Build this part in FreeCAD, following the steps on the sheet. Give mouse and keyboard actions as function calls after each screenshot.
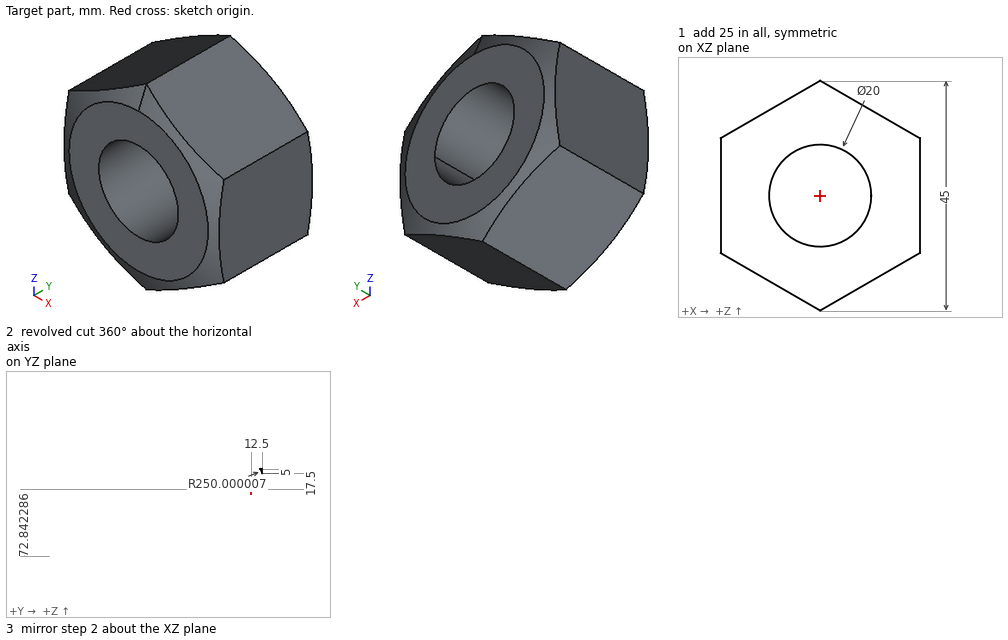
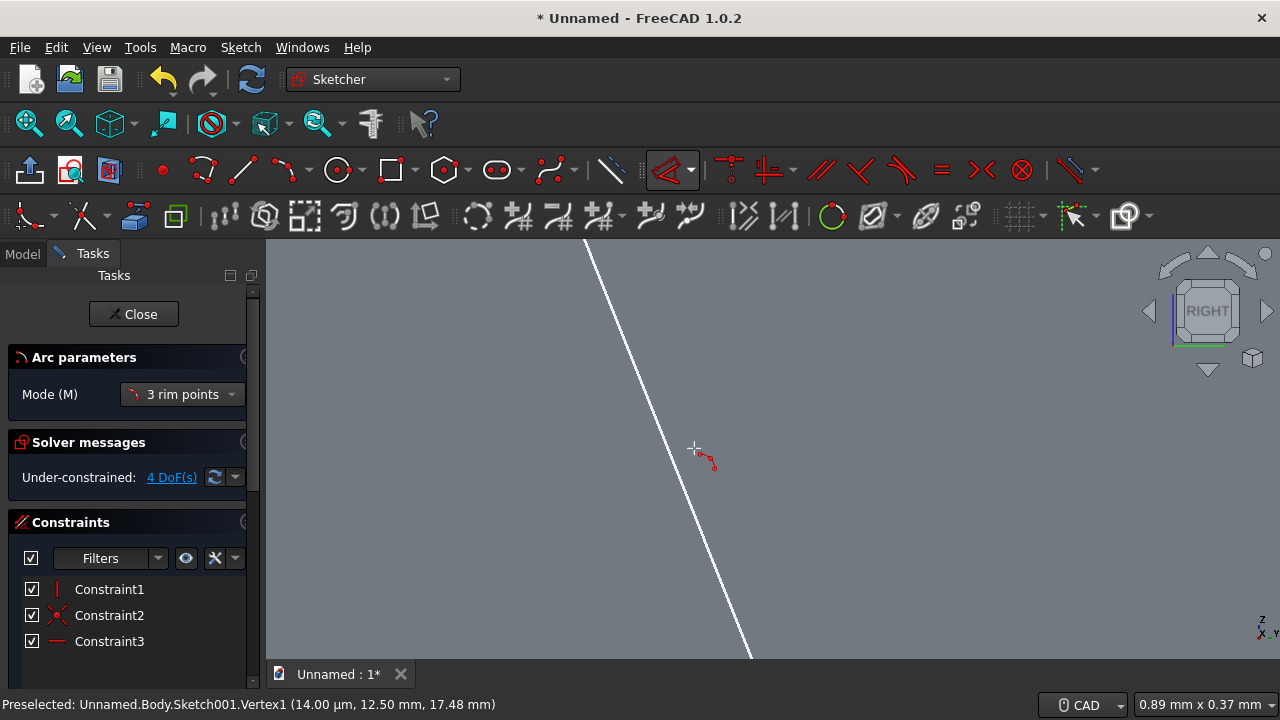
click(690, 447)
key(Escape)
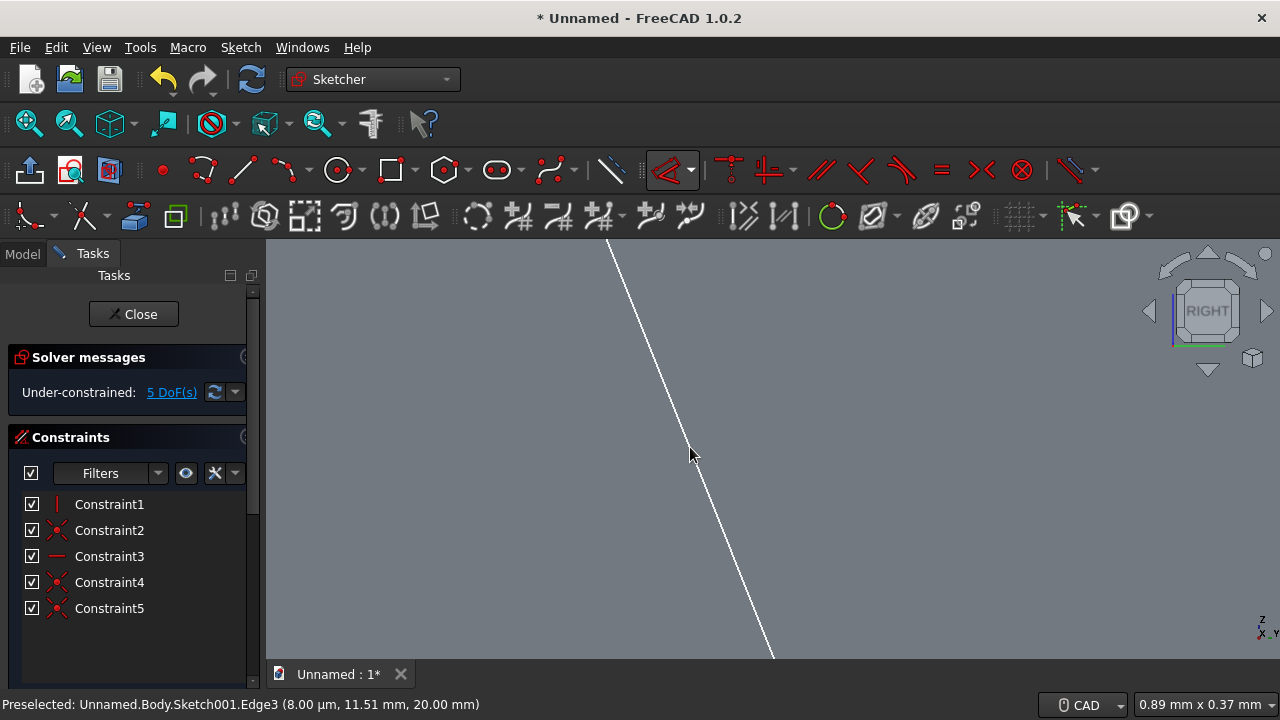
scroll(706, 449, down, 15)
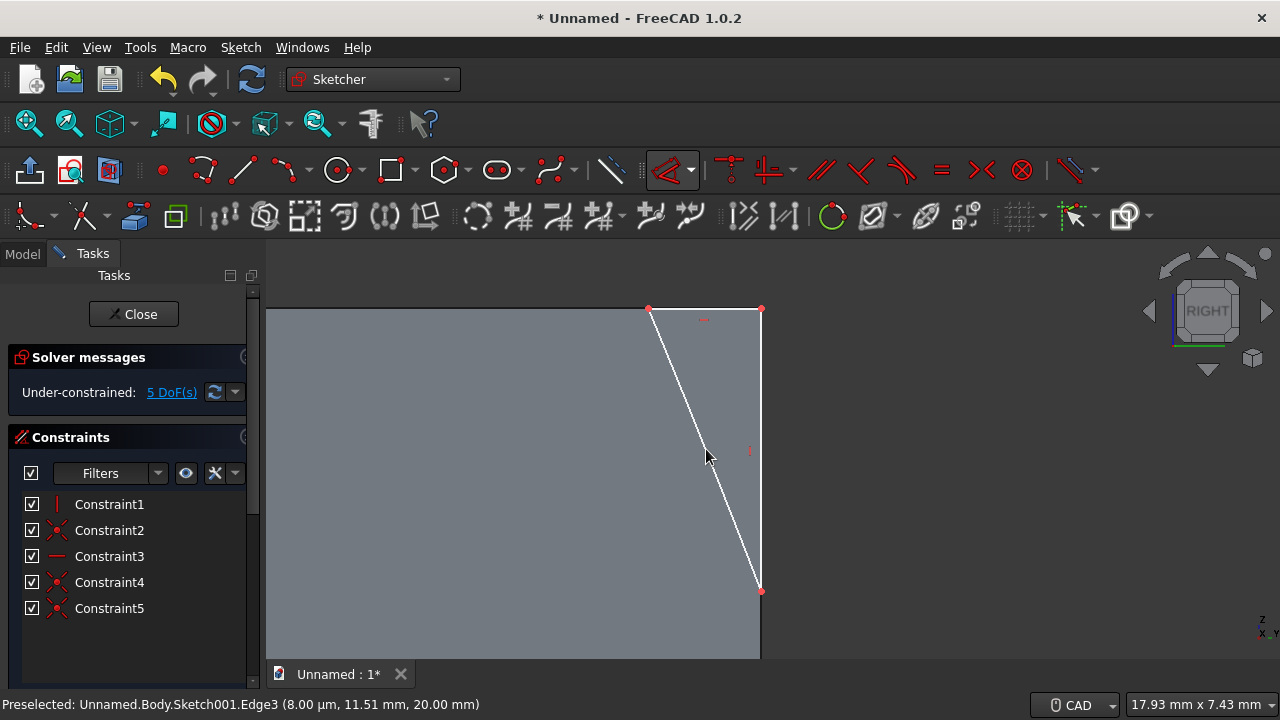
click(706, 450)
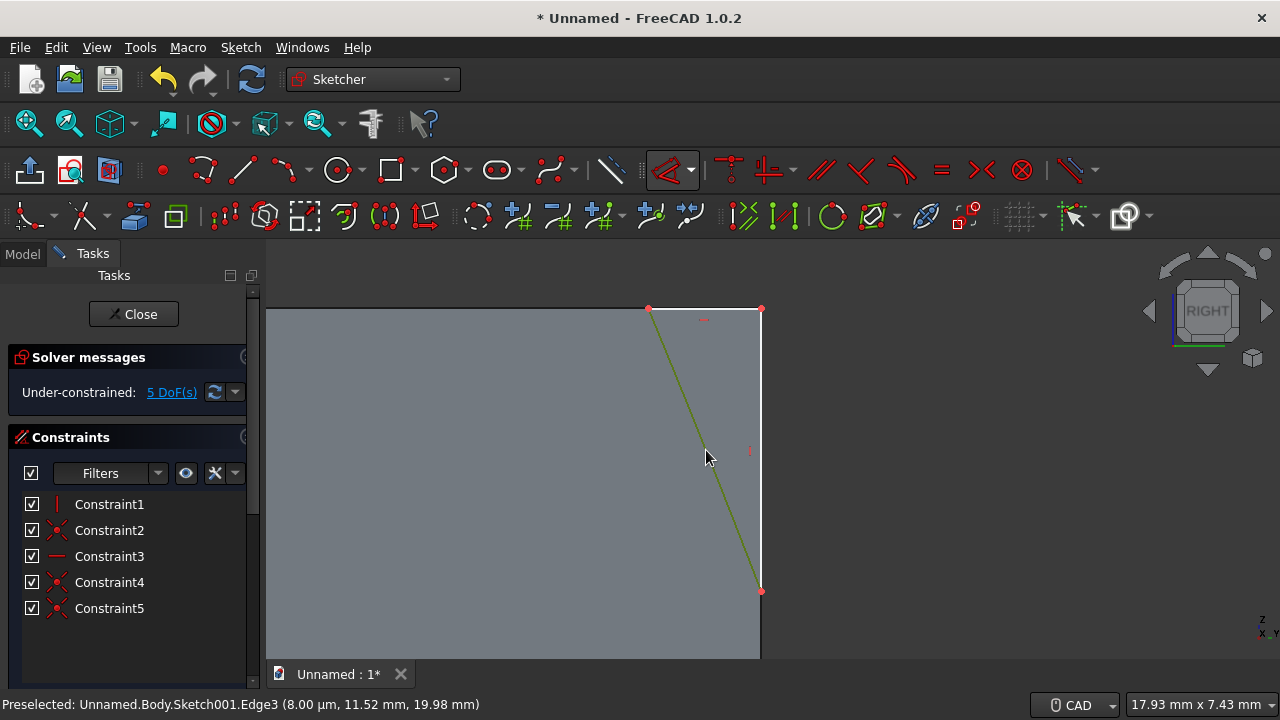
key(k)
key(r)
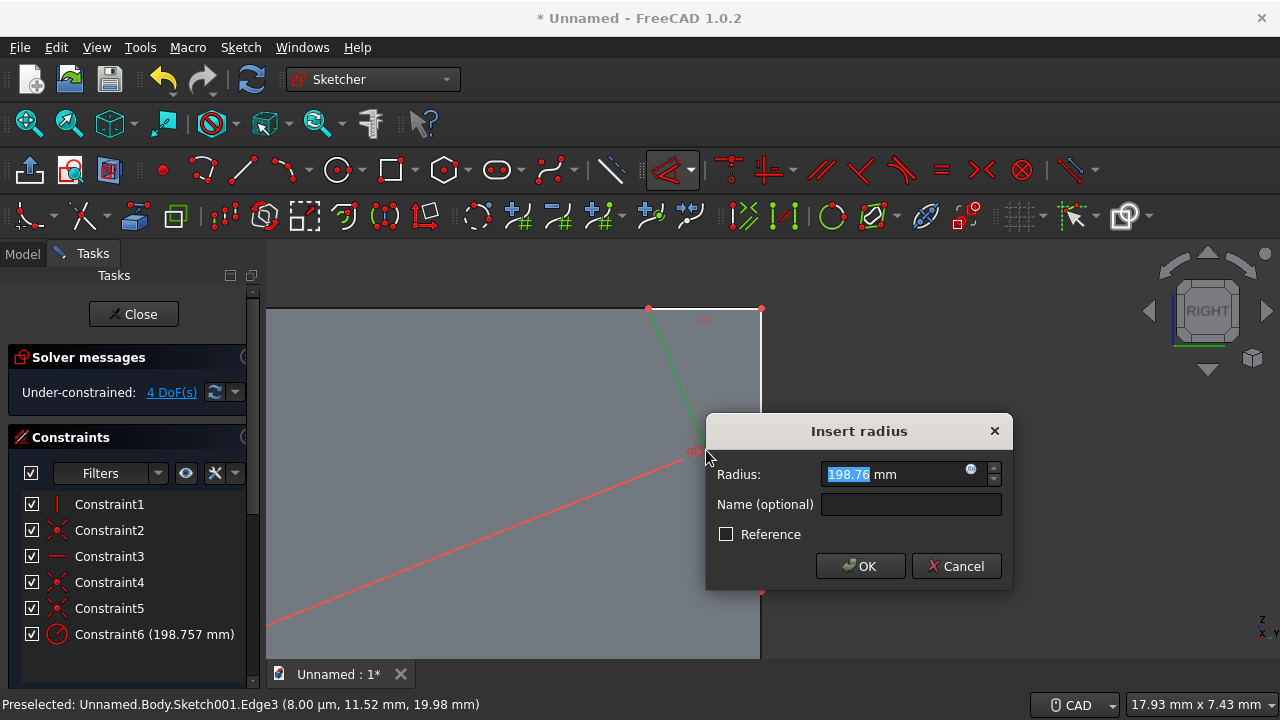
text(250.000007)
key(Return)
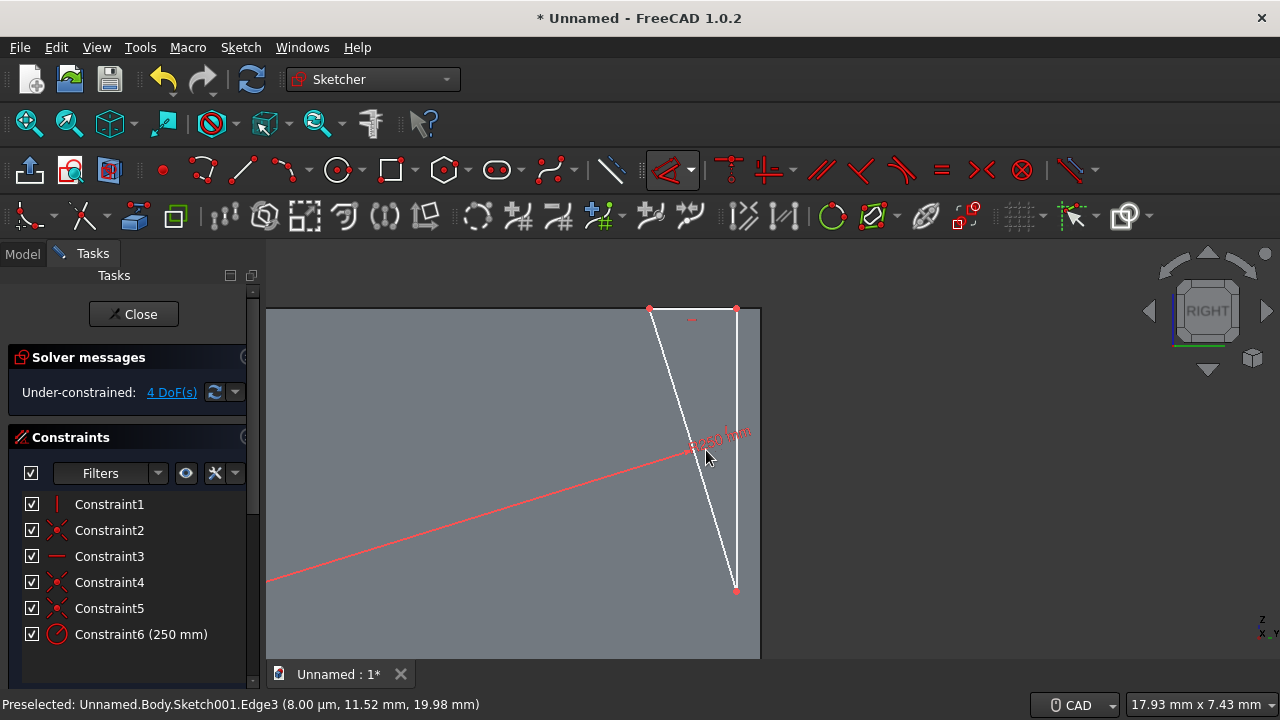
click(737, 507)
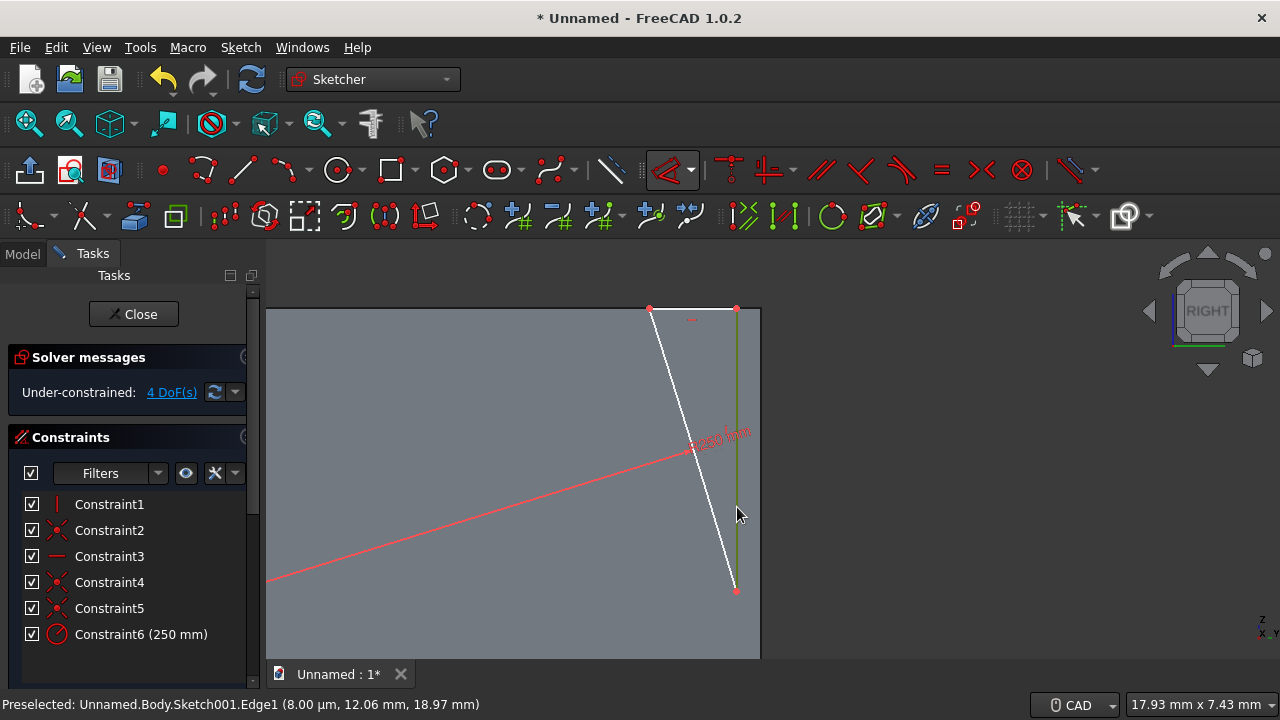
click(694, 170)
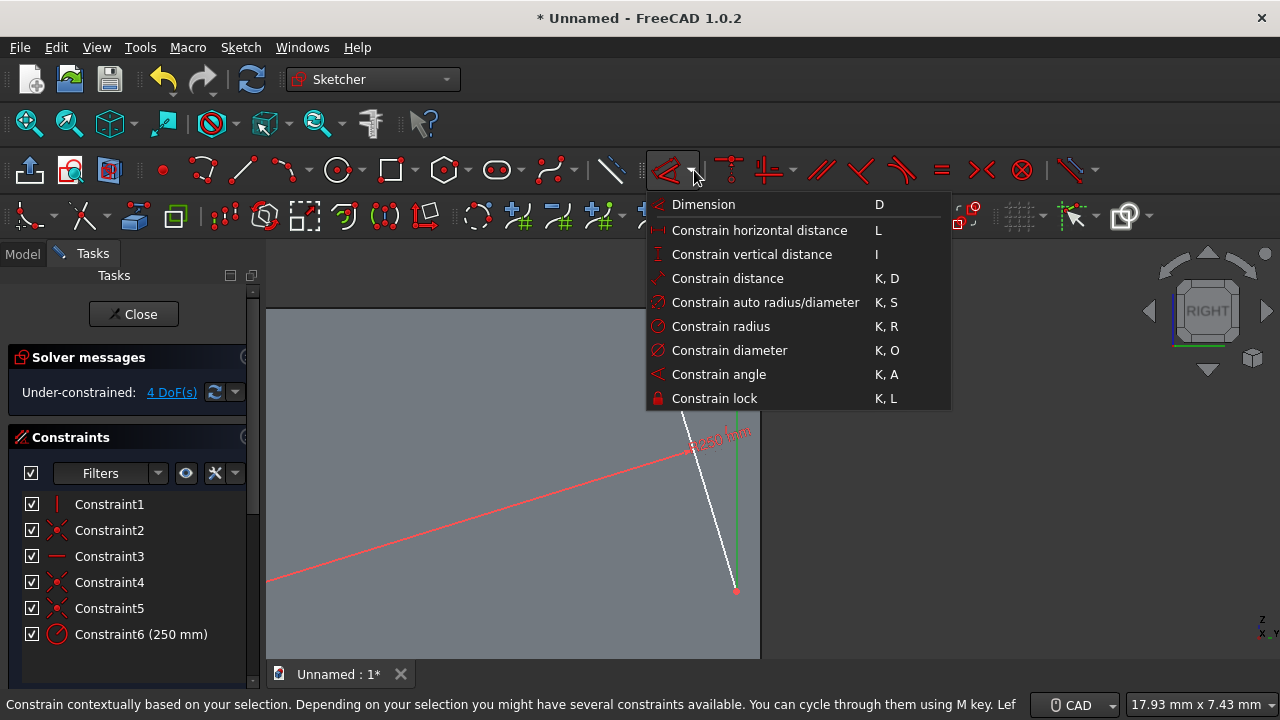
click(799, 254)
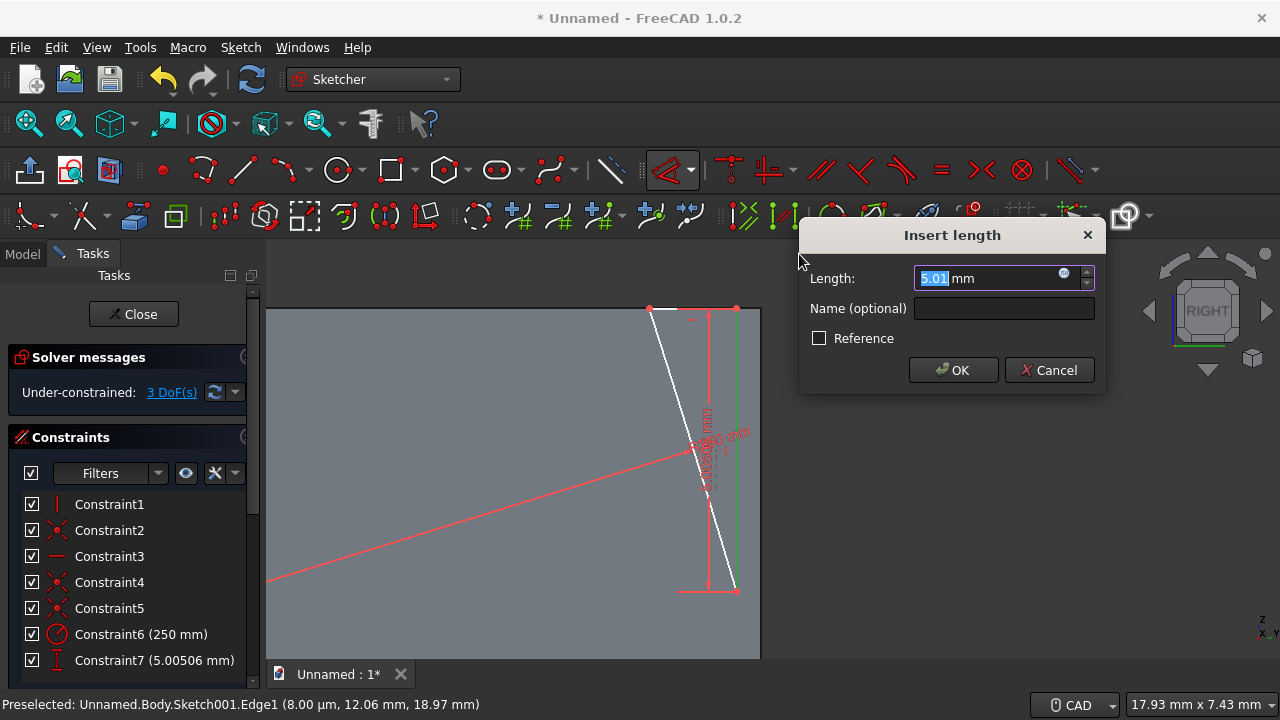
text(5)
key(Return)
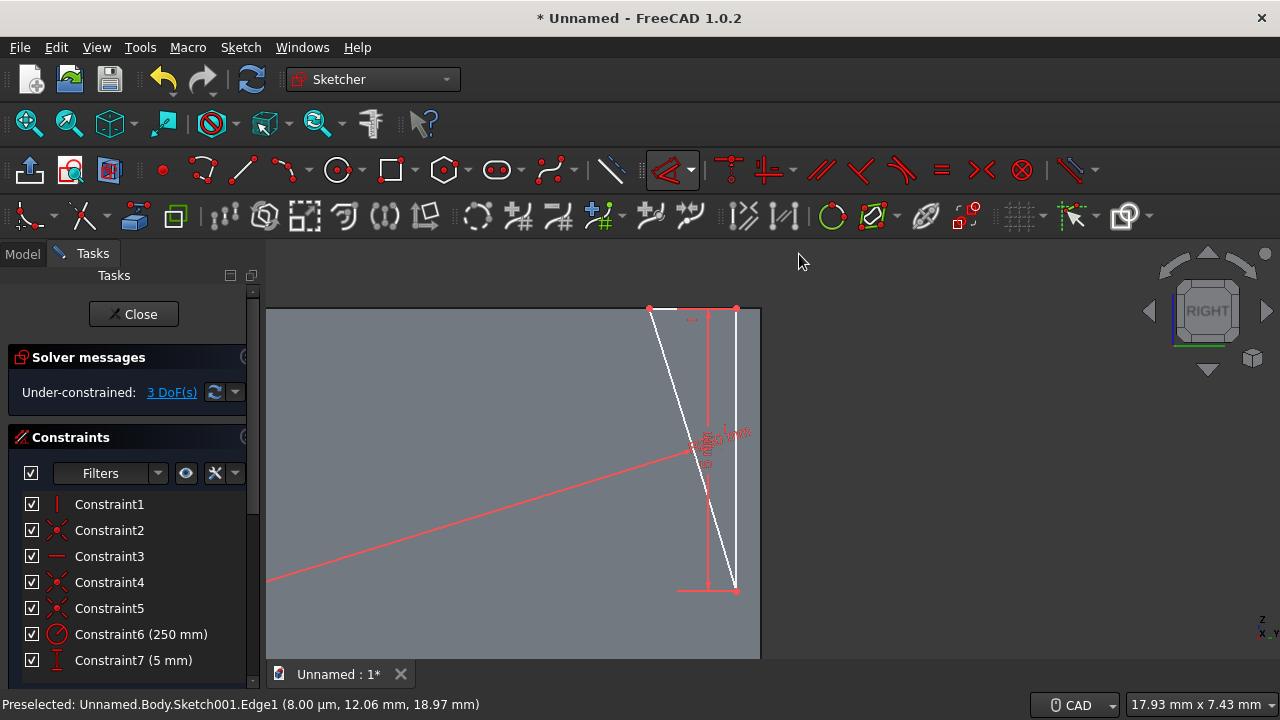
click(736, 591)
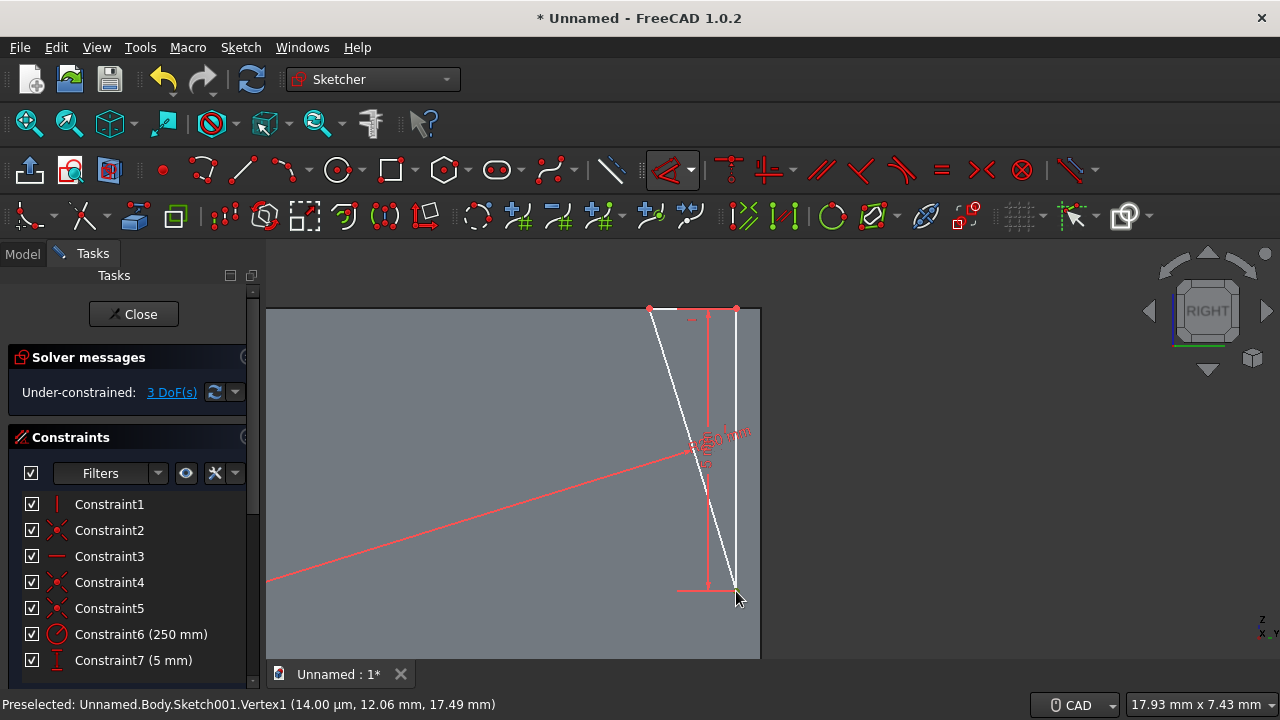
key(l)